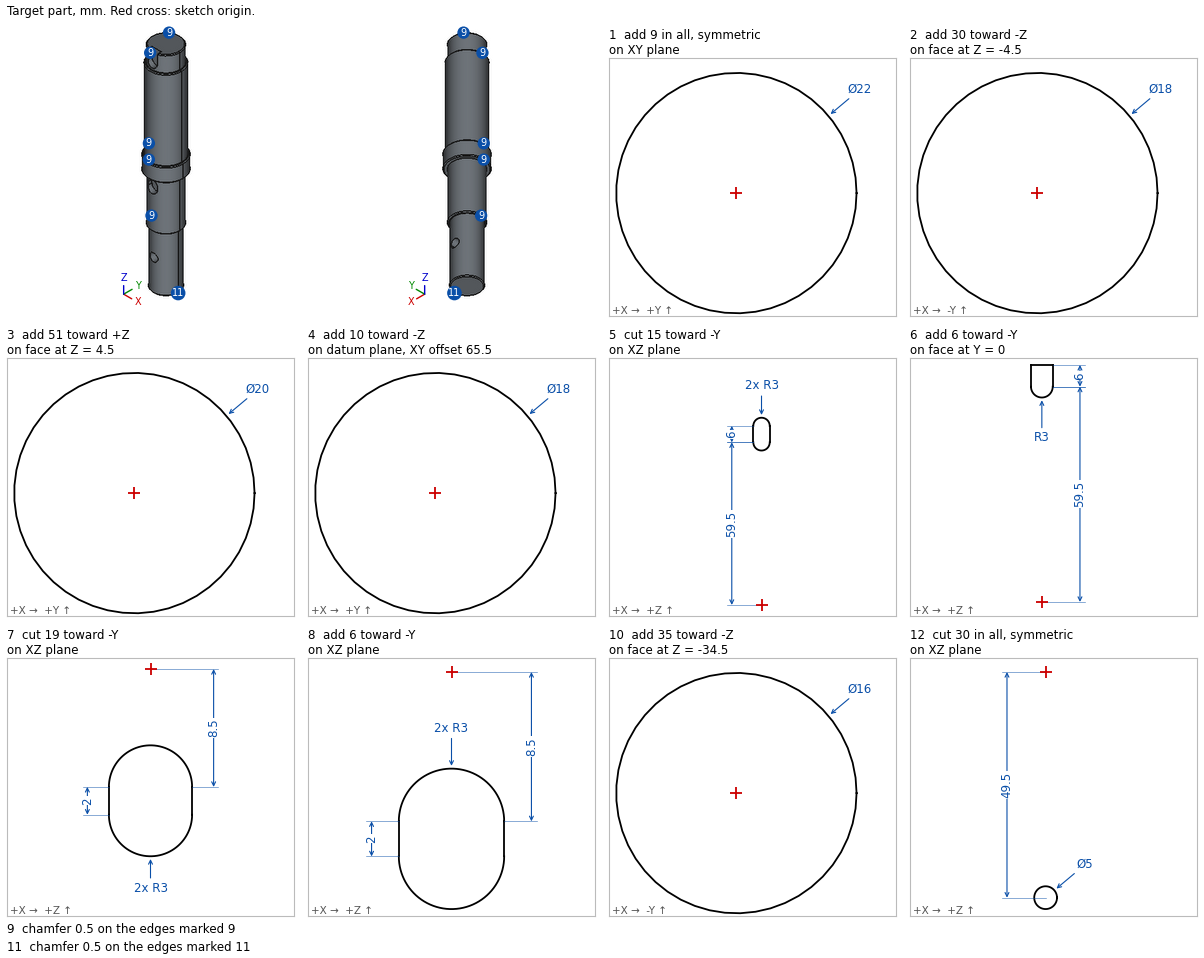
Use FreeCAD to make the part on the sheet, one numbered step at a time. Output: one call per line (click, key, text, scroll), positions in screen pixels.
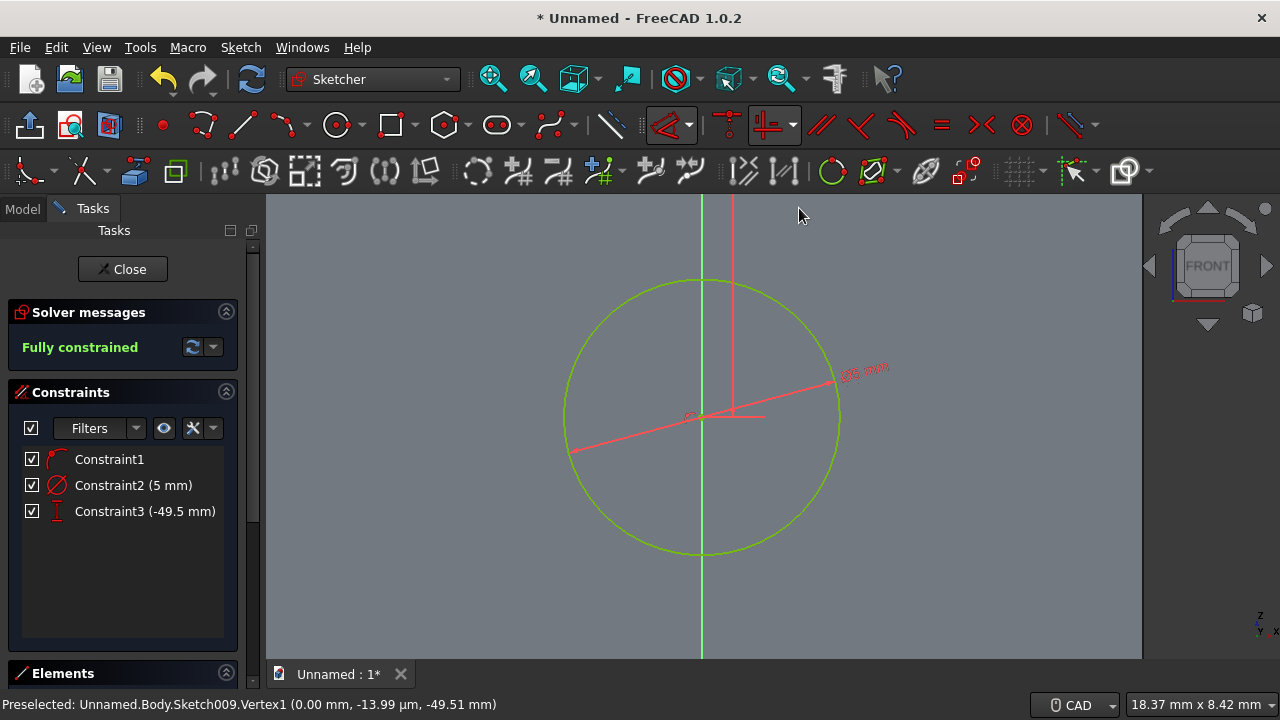
click(123, 269)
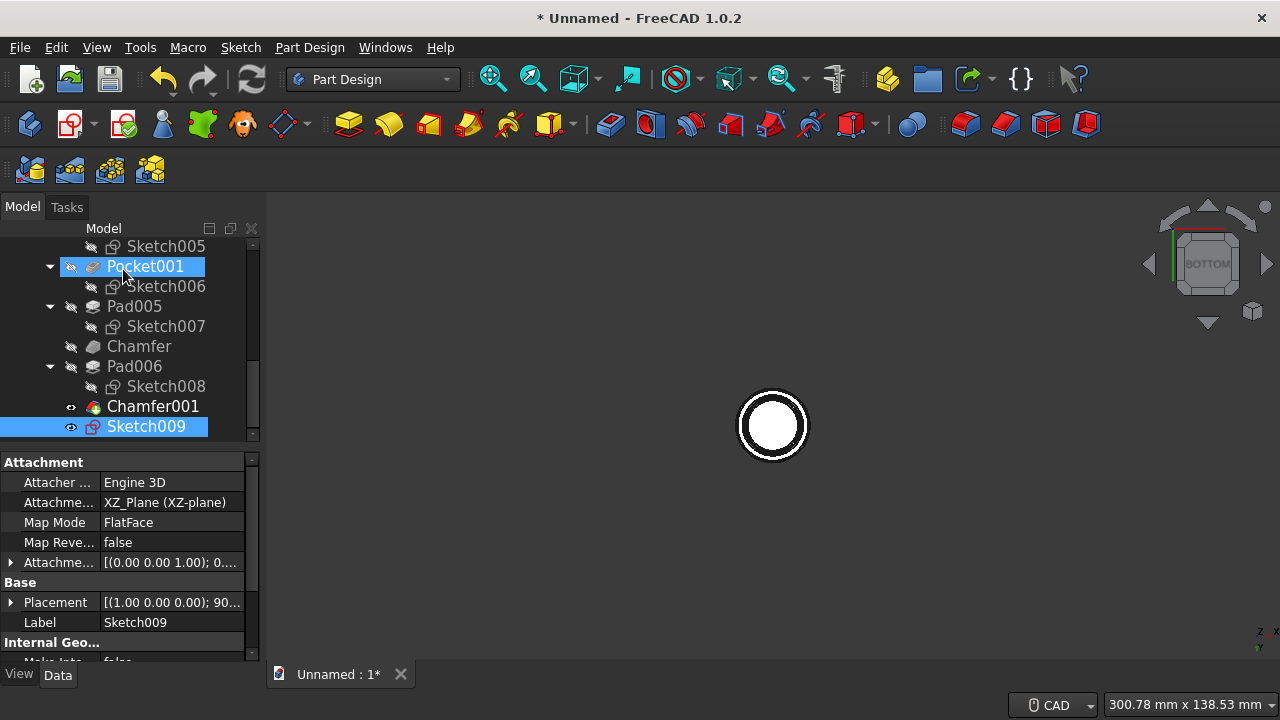
click(612, 124)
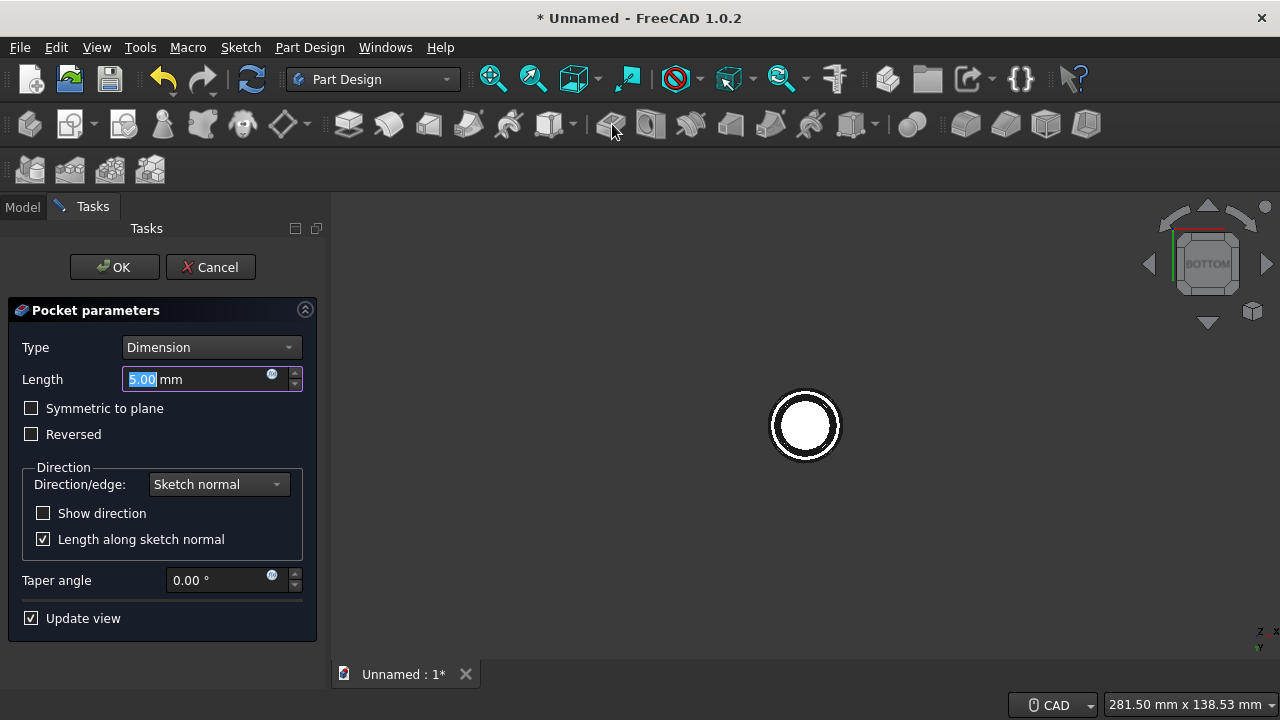
text(30)
key(Tab)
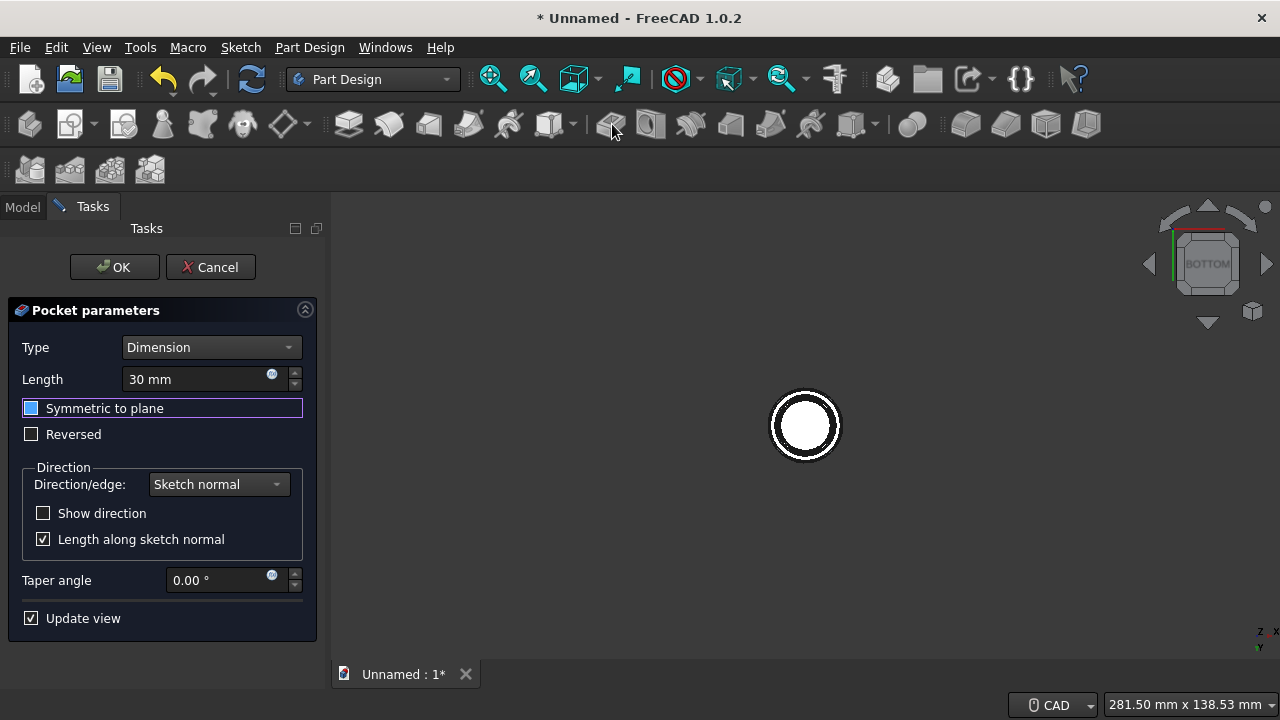
click(30, 408)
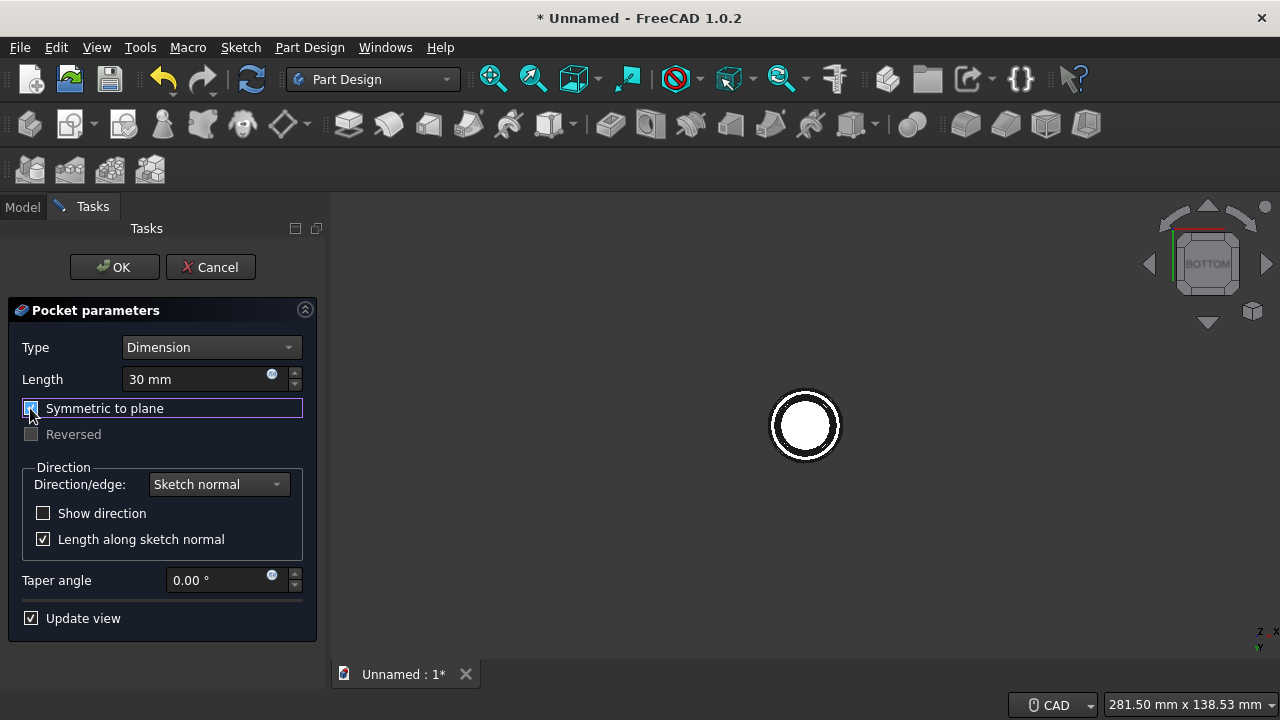
click(115, 267)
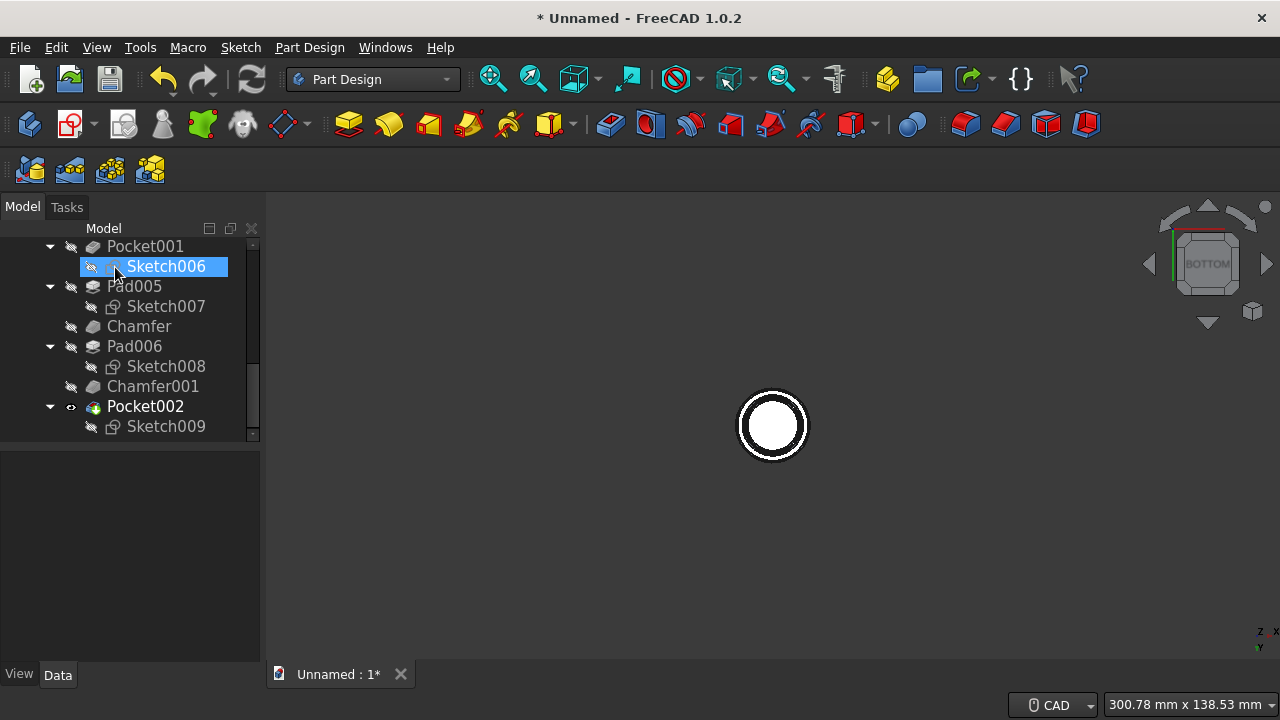
key(0)